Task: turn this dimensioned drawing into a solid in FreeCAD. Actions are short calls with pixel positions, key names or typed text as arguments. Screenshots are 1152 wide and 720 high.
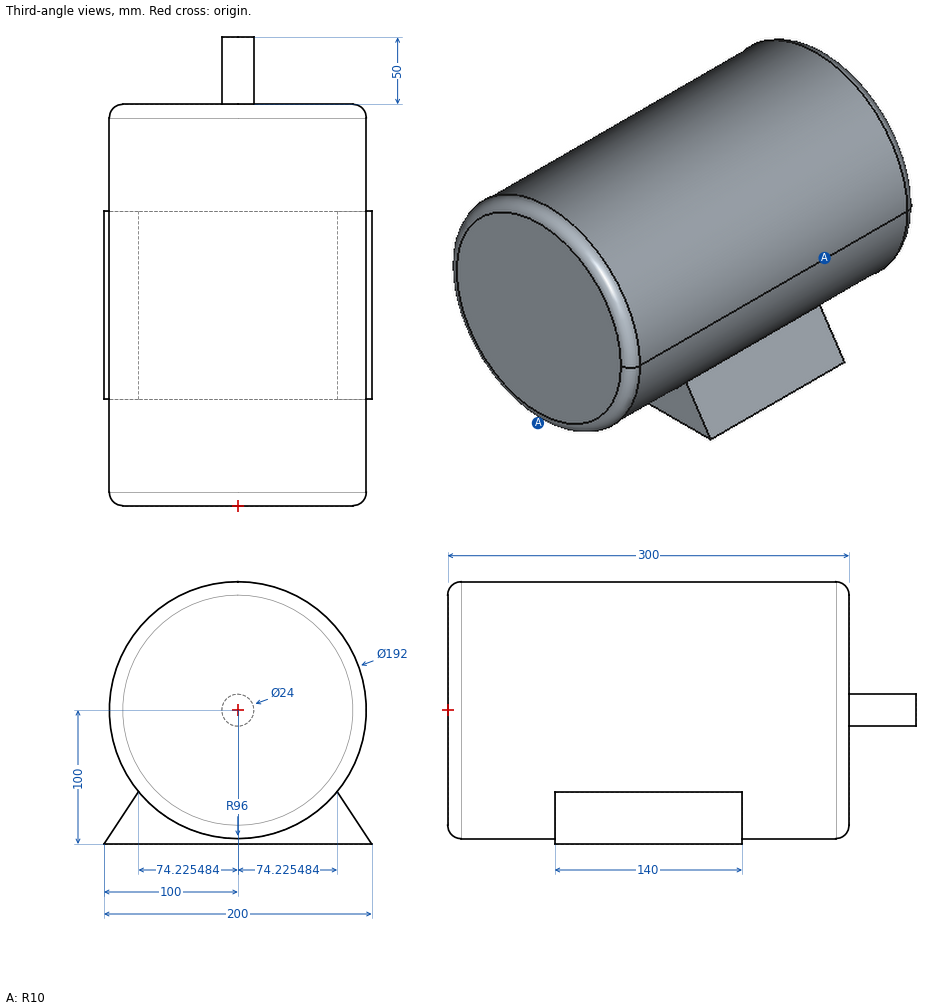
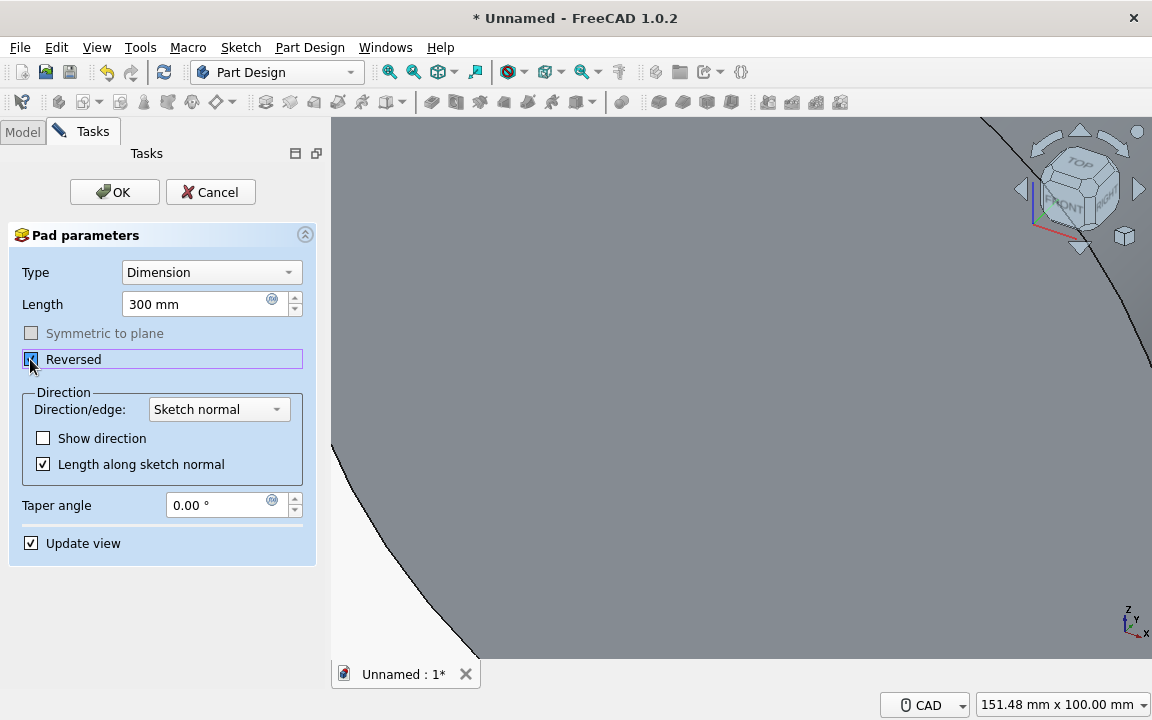
click(115, 192)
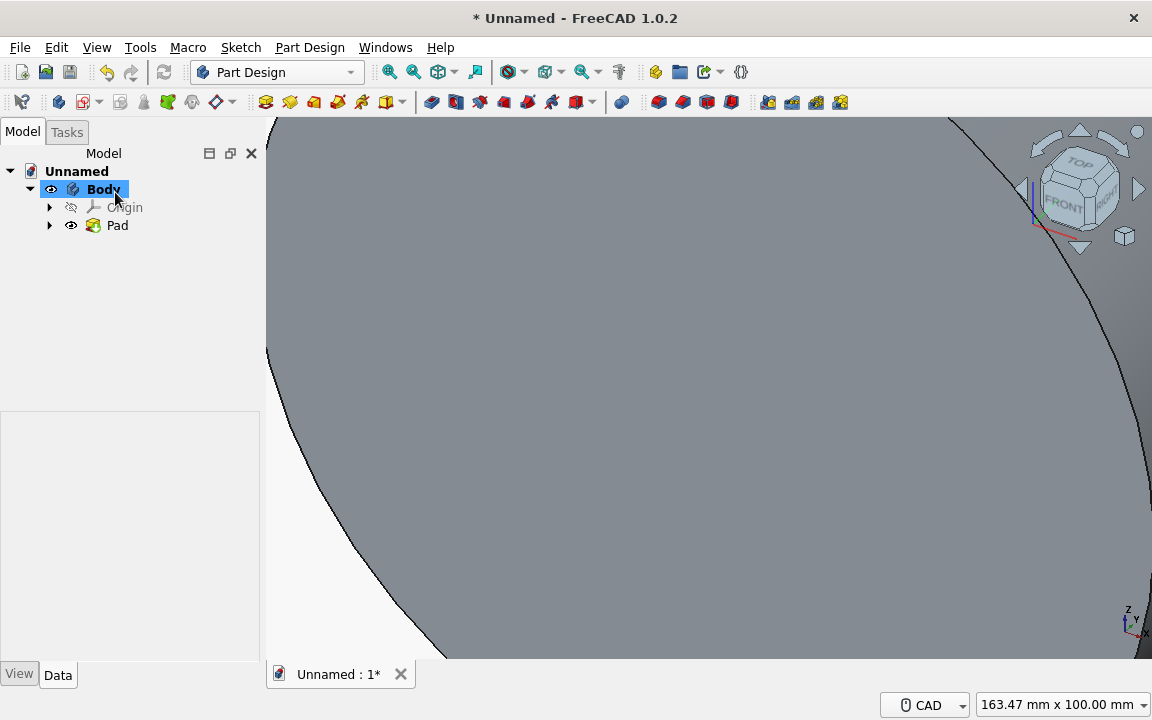
click(390, 72)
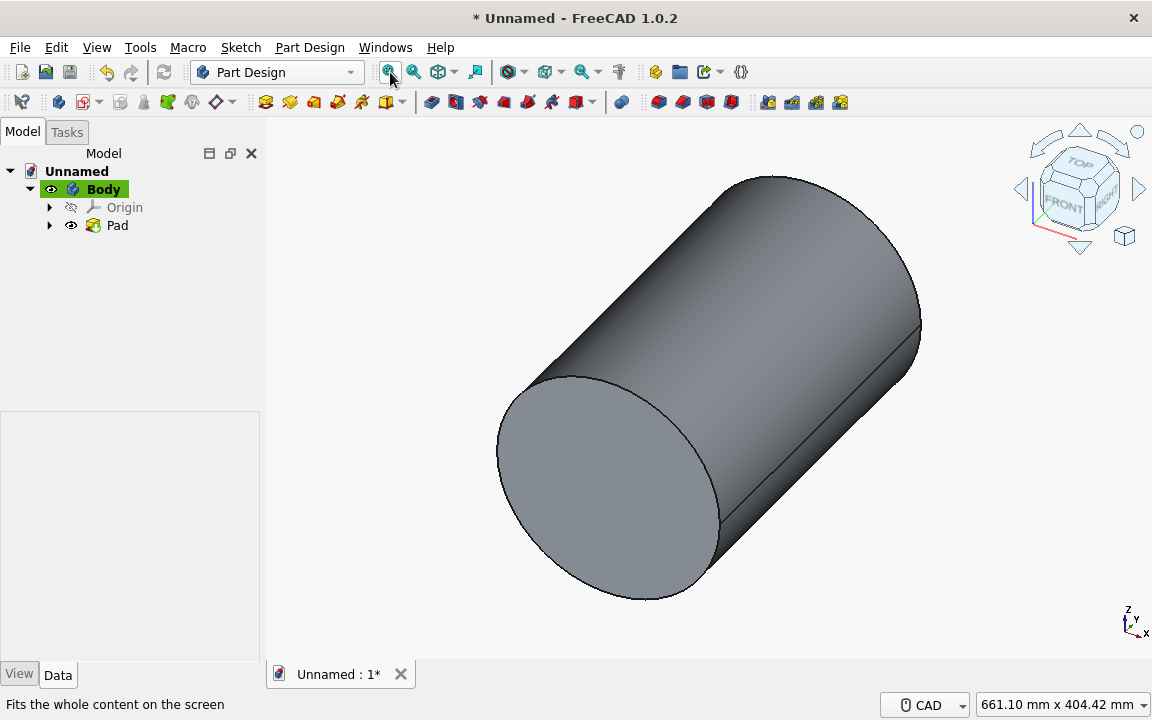
key(4)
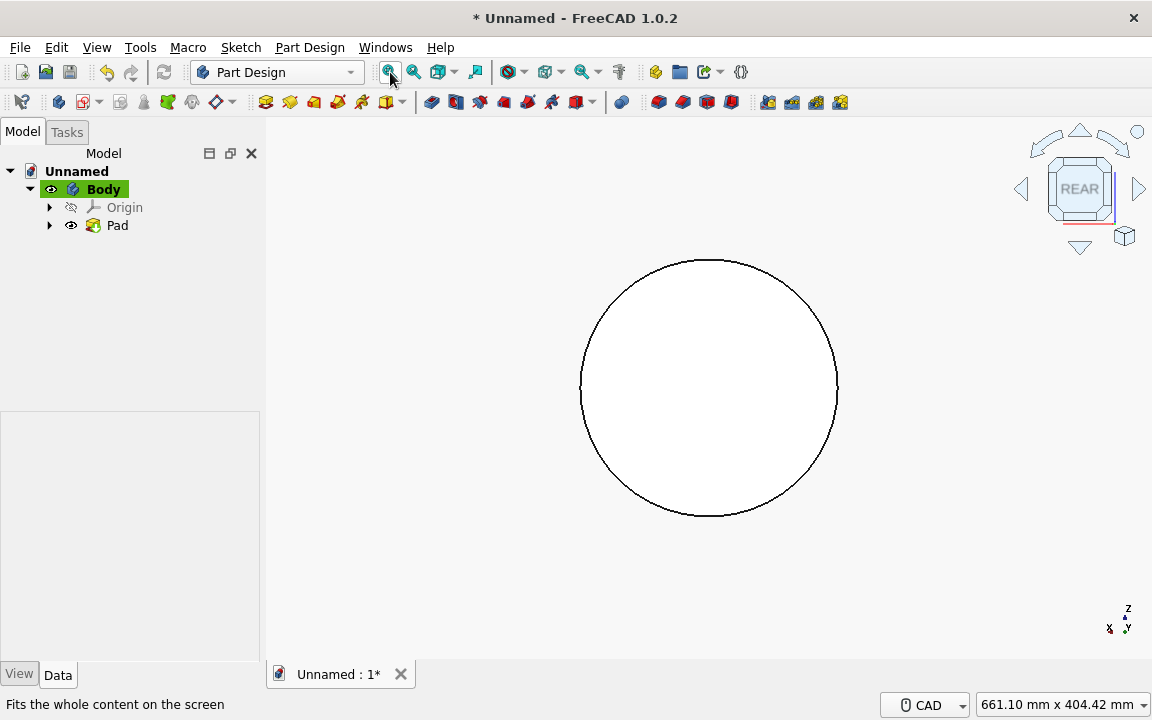
click(709, 387)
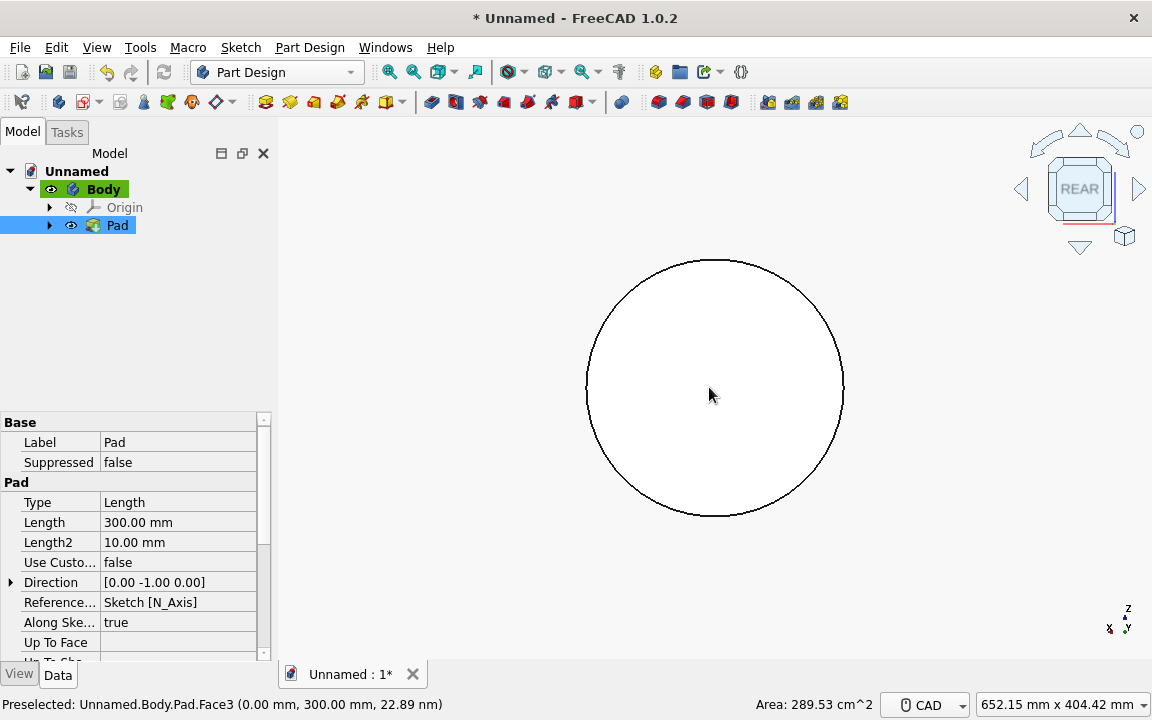
click(84, 102)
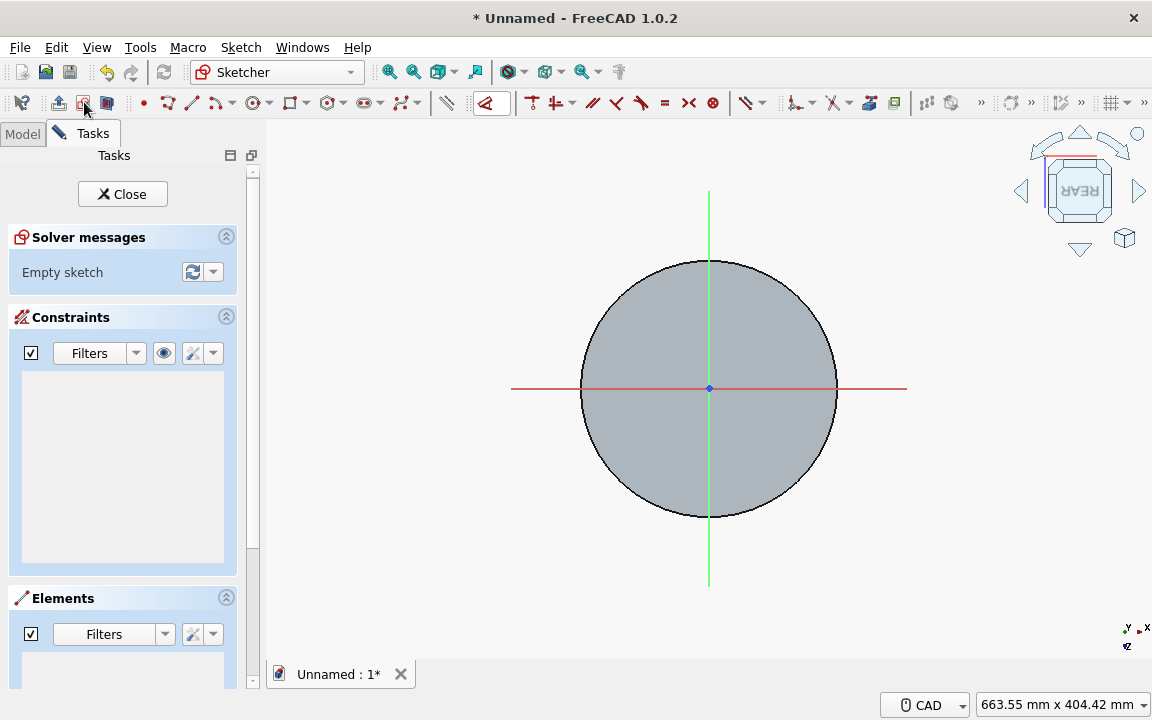
scroll(716, 389, up, 12)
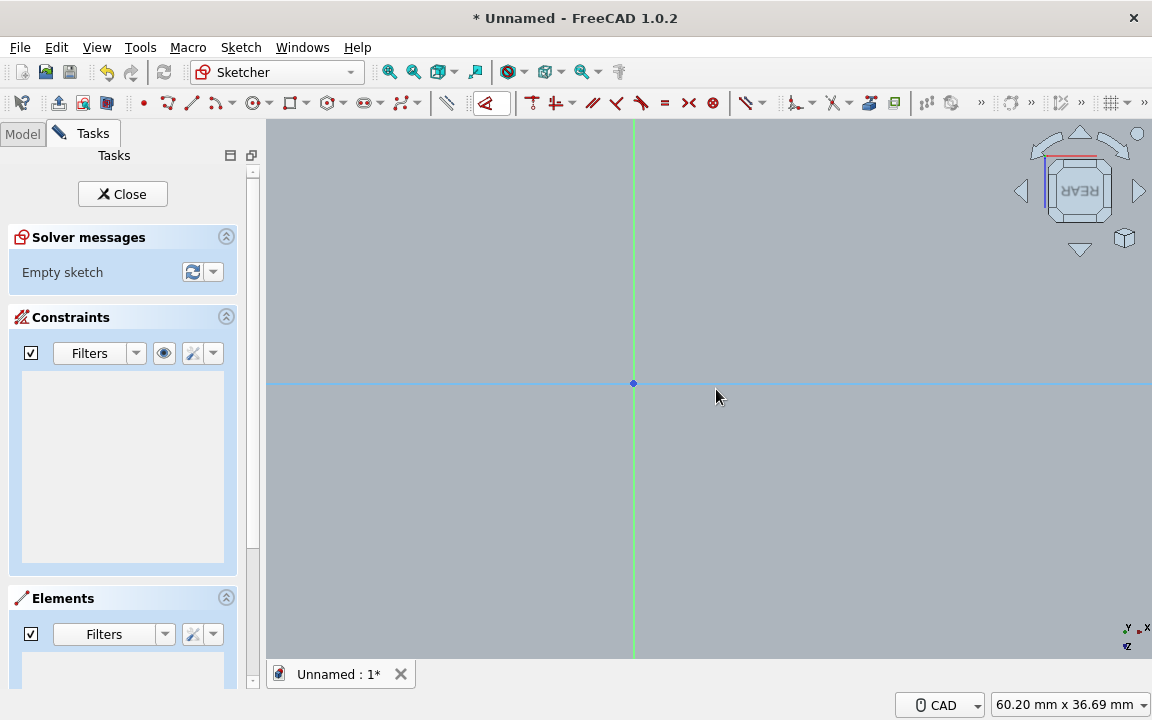
key(g)
key(c)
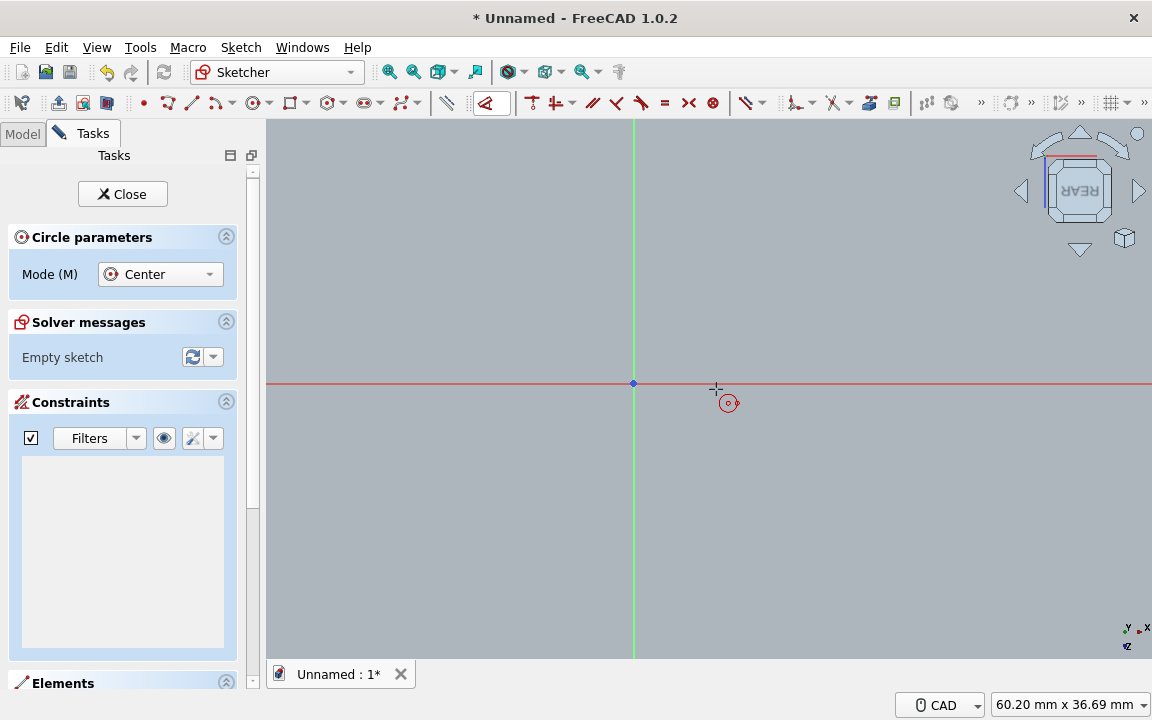
click(634, 384)
move(759, 259)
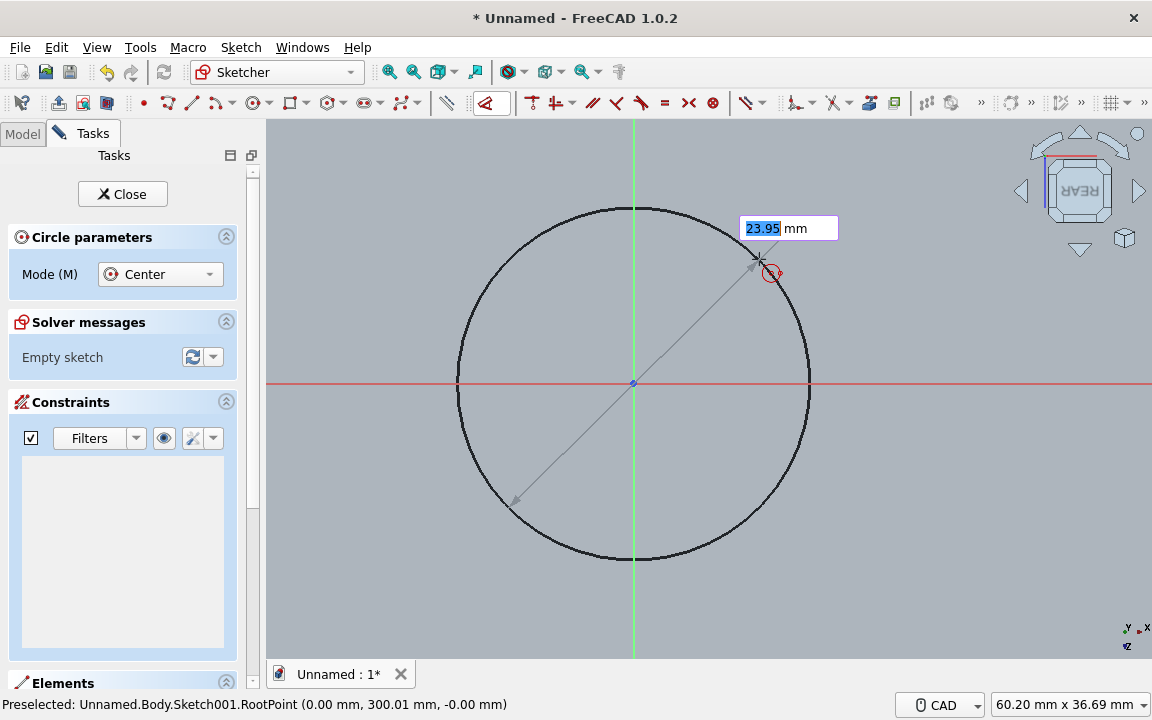
text(24)
key(Return)
key(Escape)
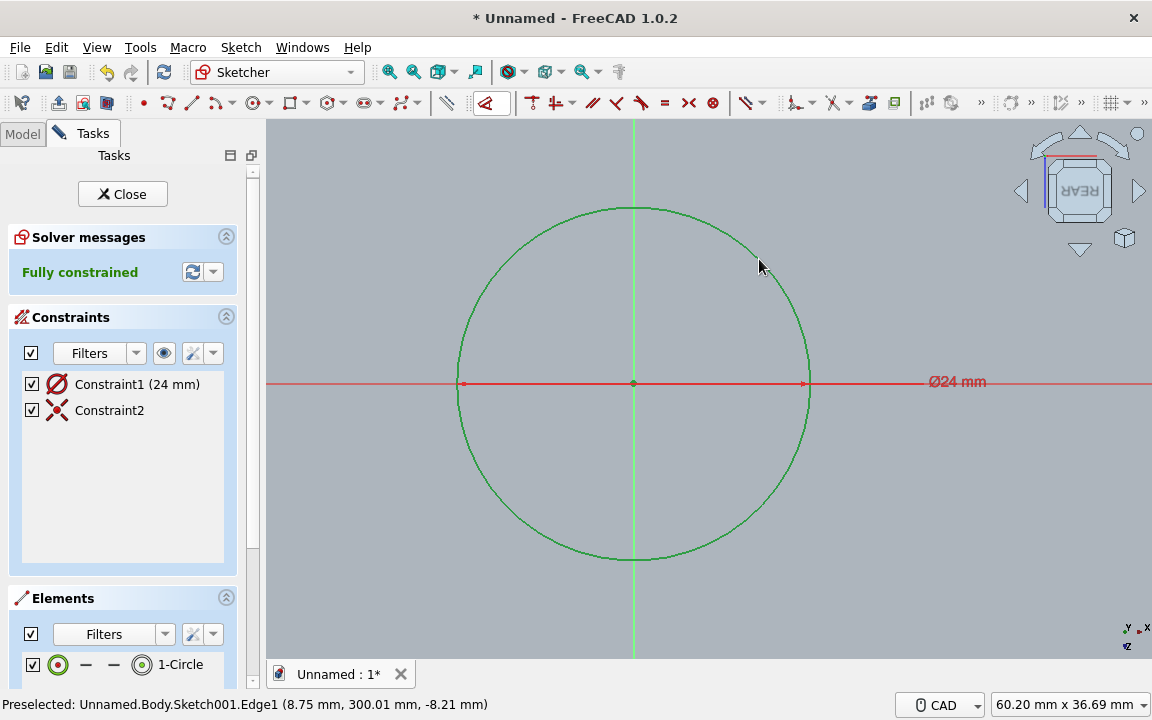
click(123, 194)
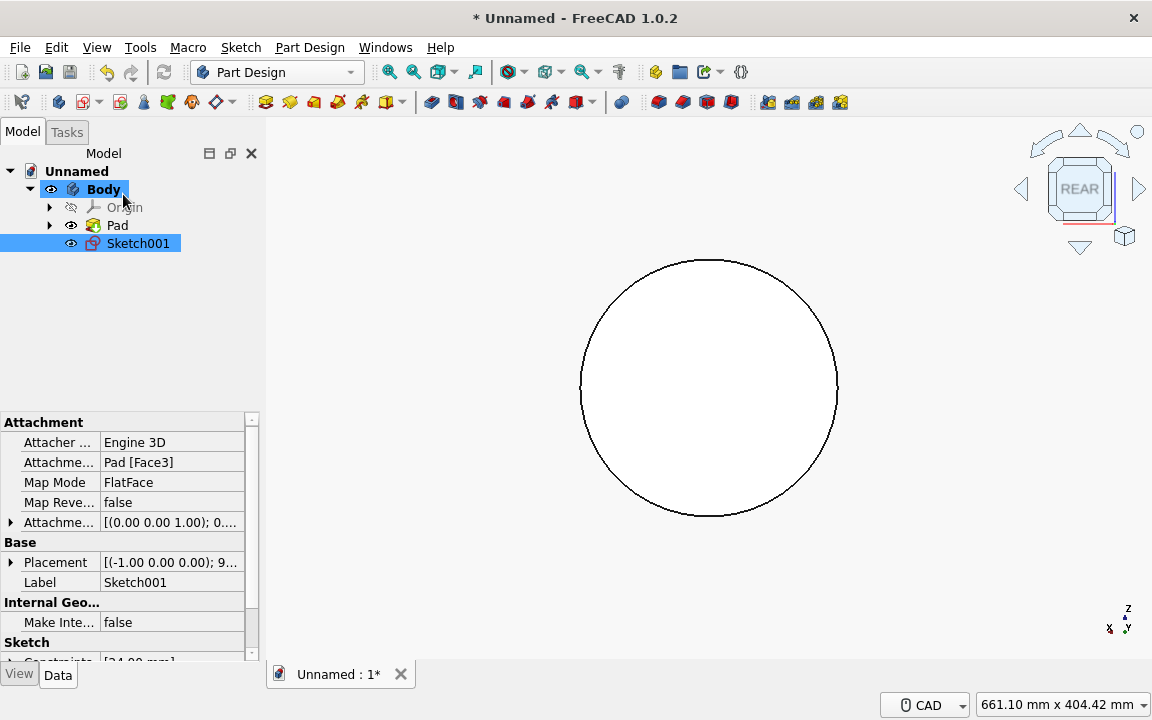
click(266, 102)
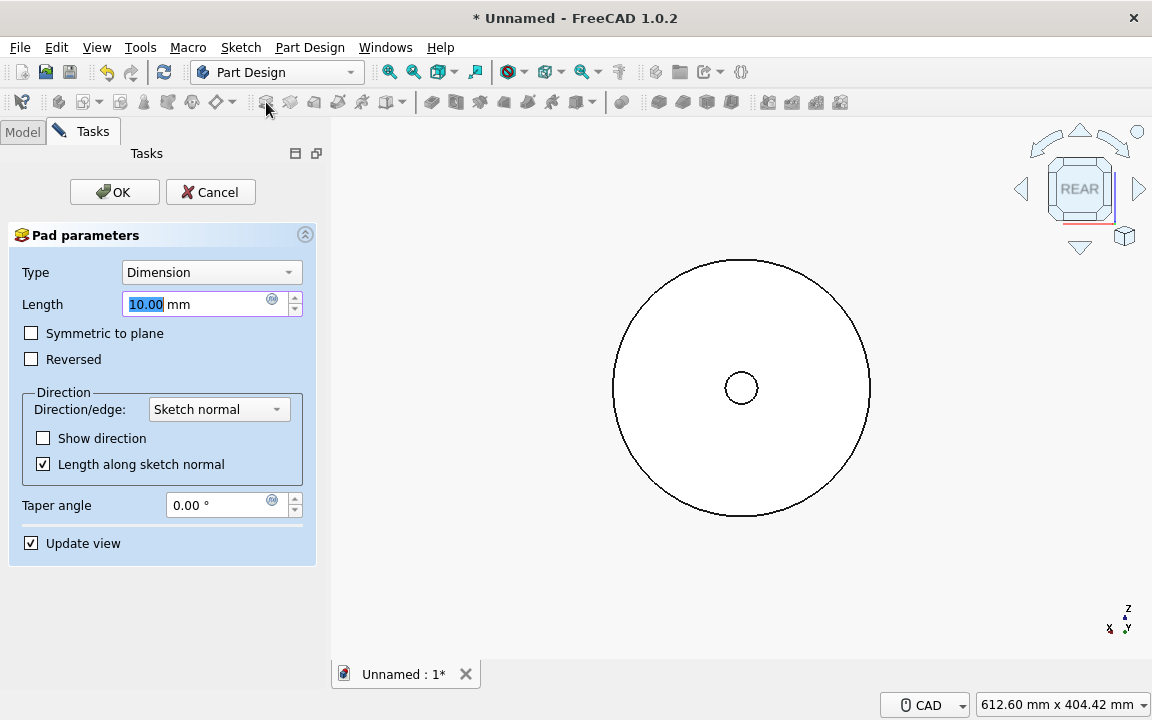
text(50)
key(Tab)